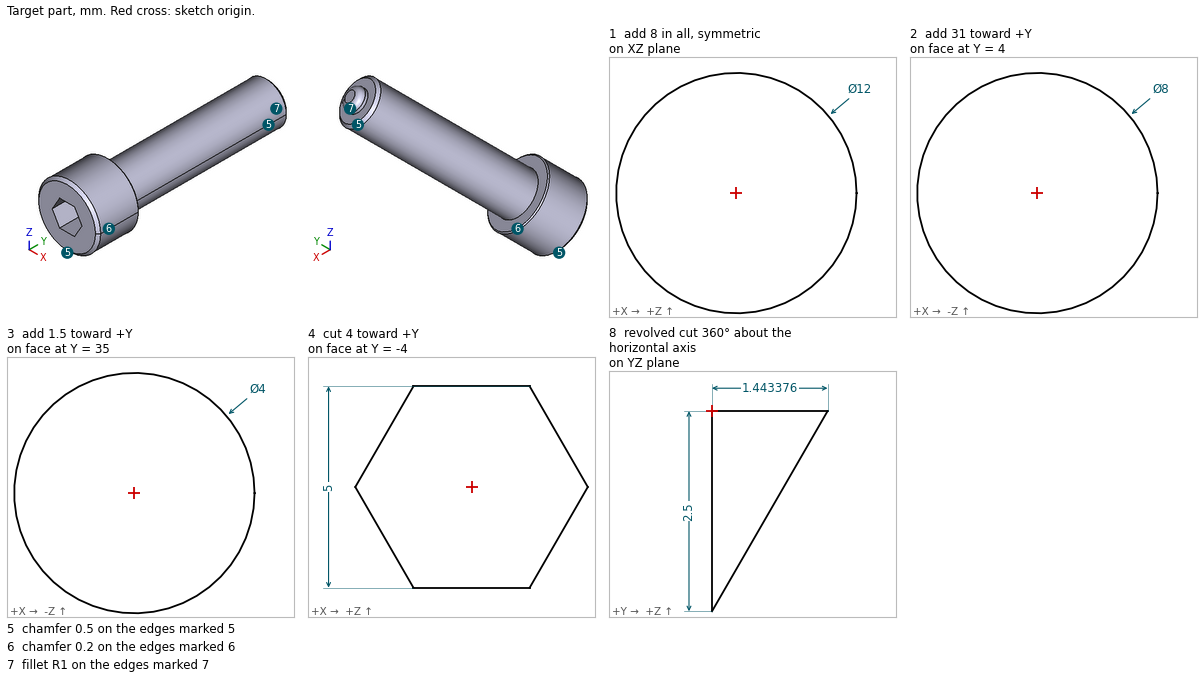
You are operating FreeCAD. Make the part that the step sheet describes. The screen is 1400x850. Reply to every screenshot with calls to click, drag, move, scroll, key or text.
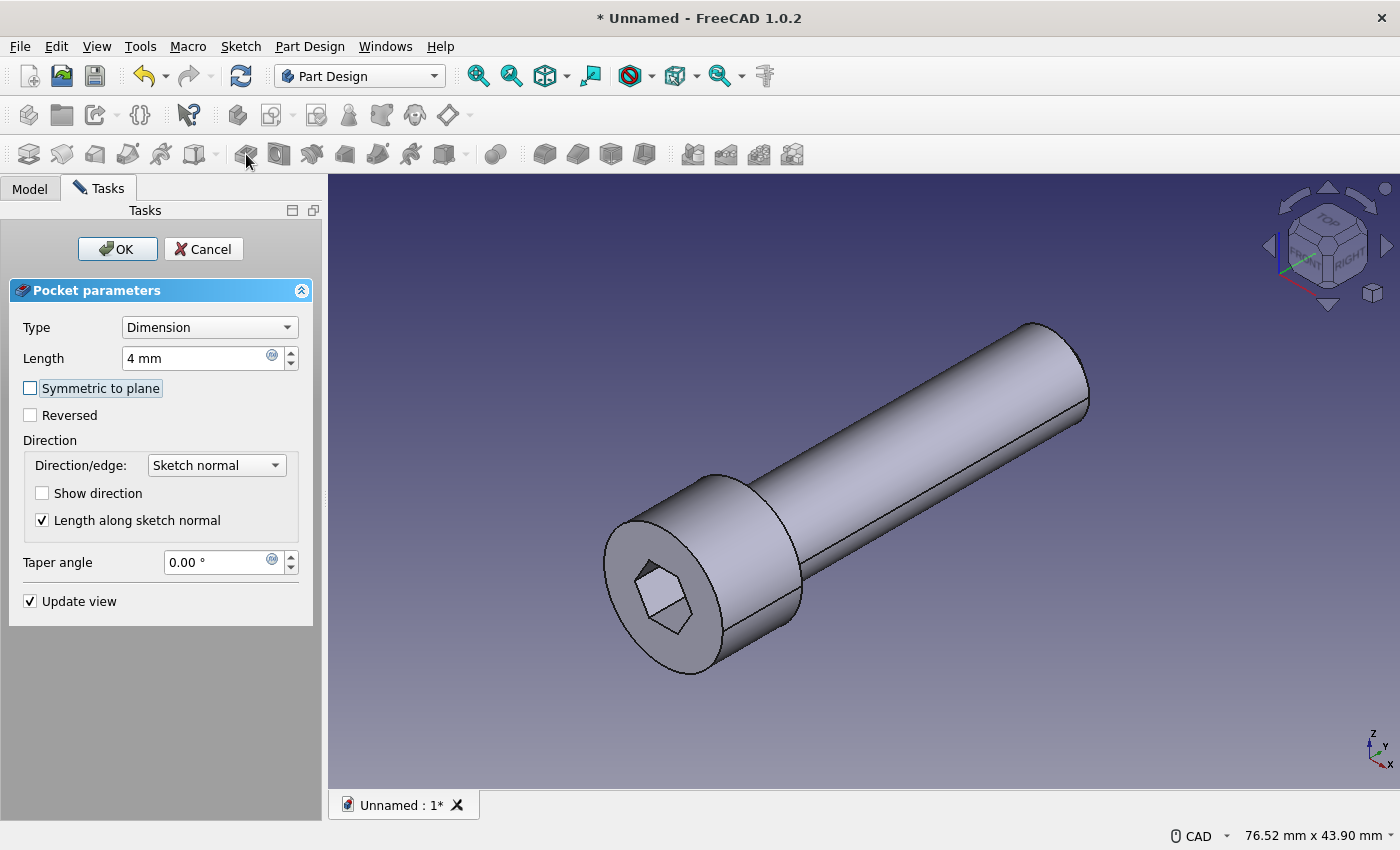
click(118, 249)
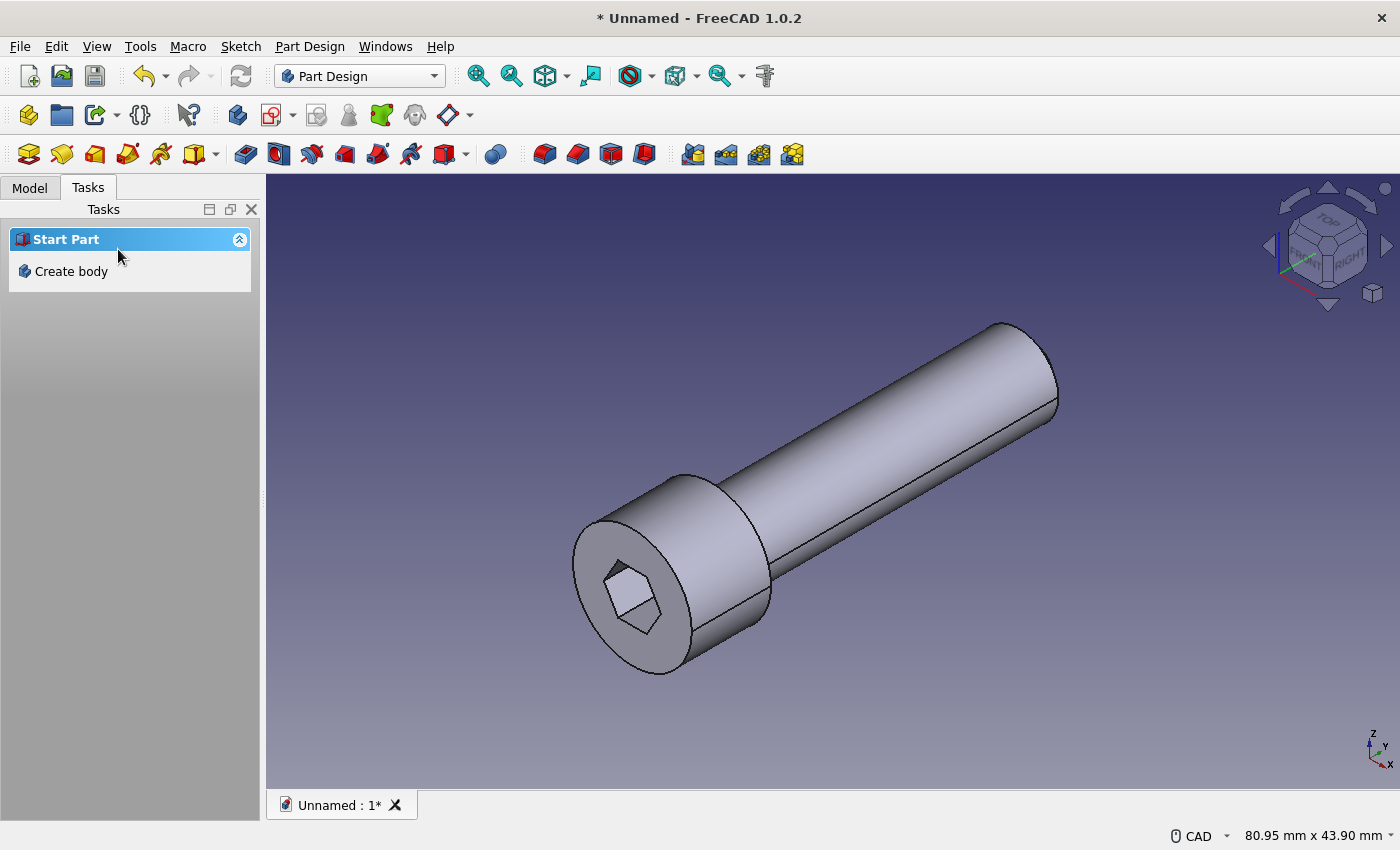
click(584, 528)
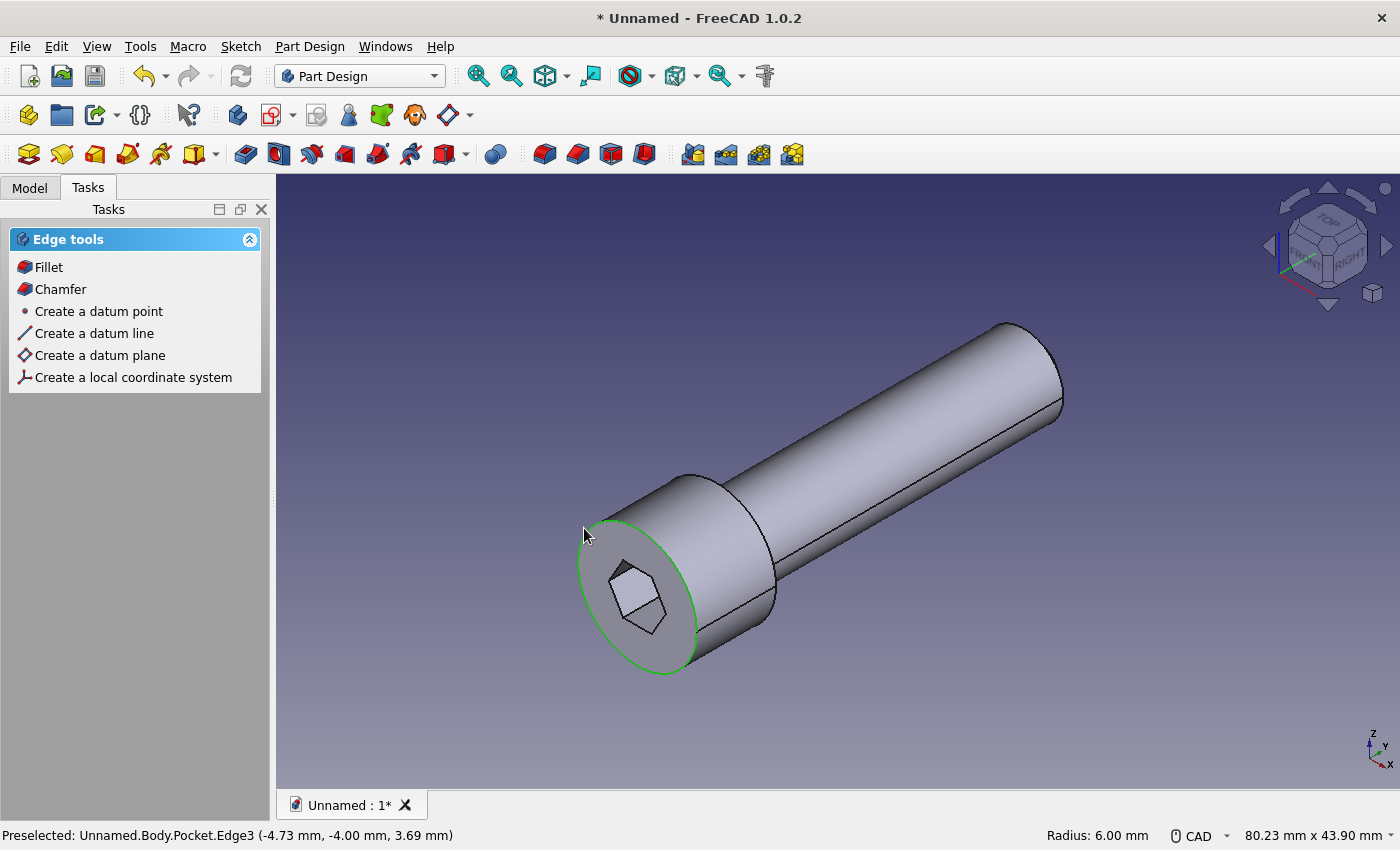
key(2)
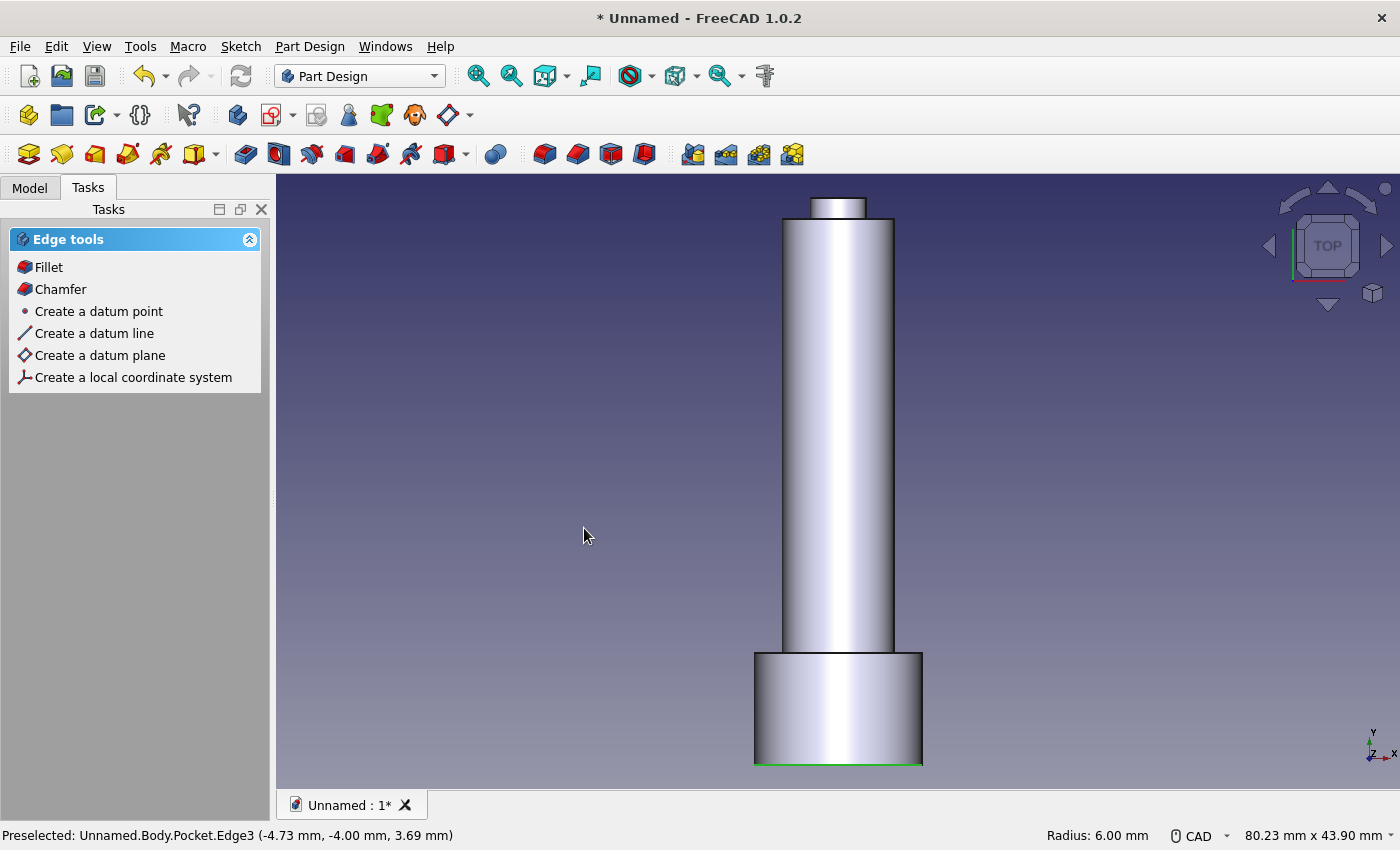
click(793, 218, ctrl)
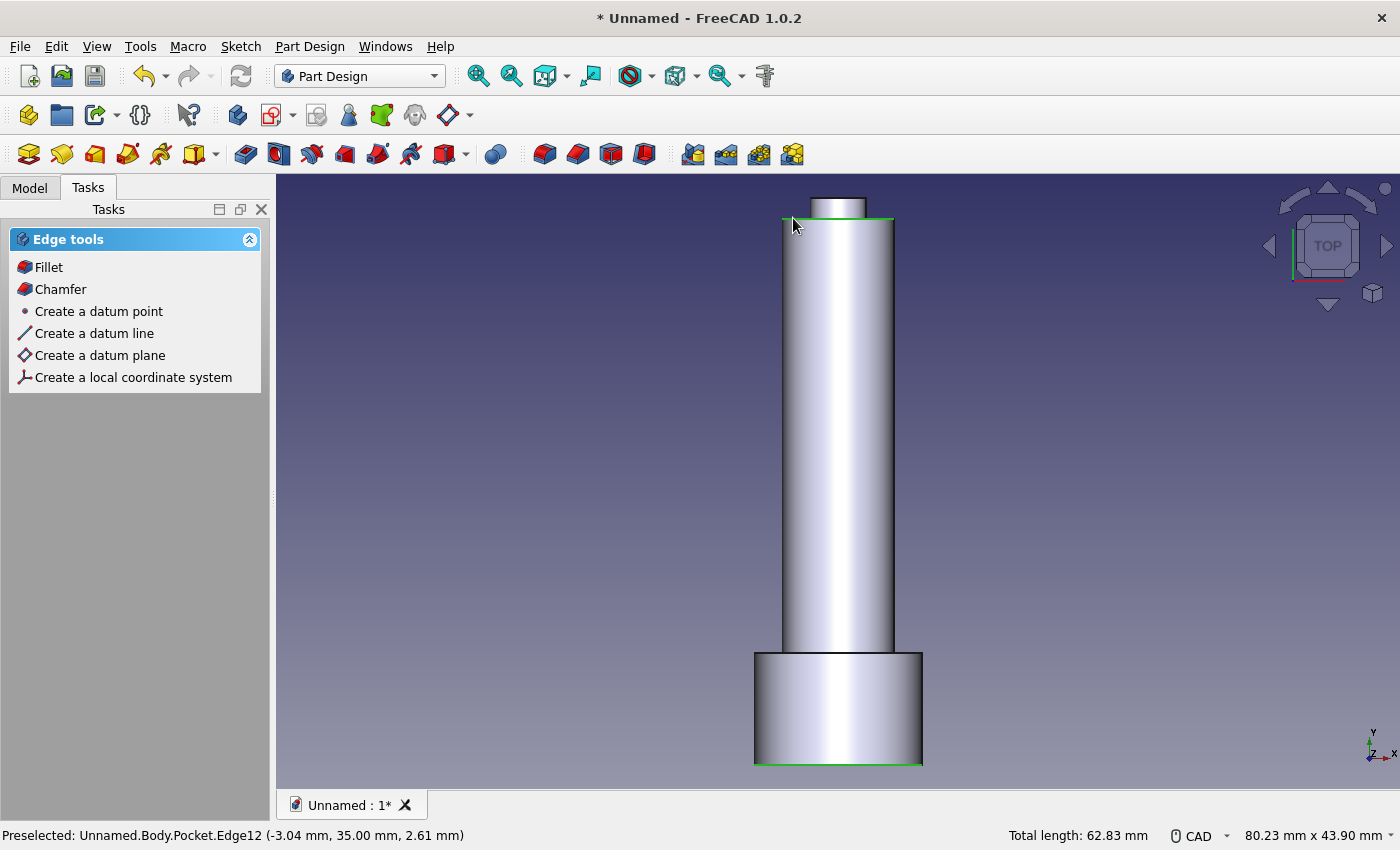
click(578, 154)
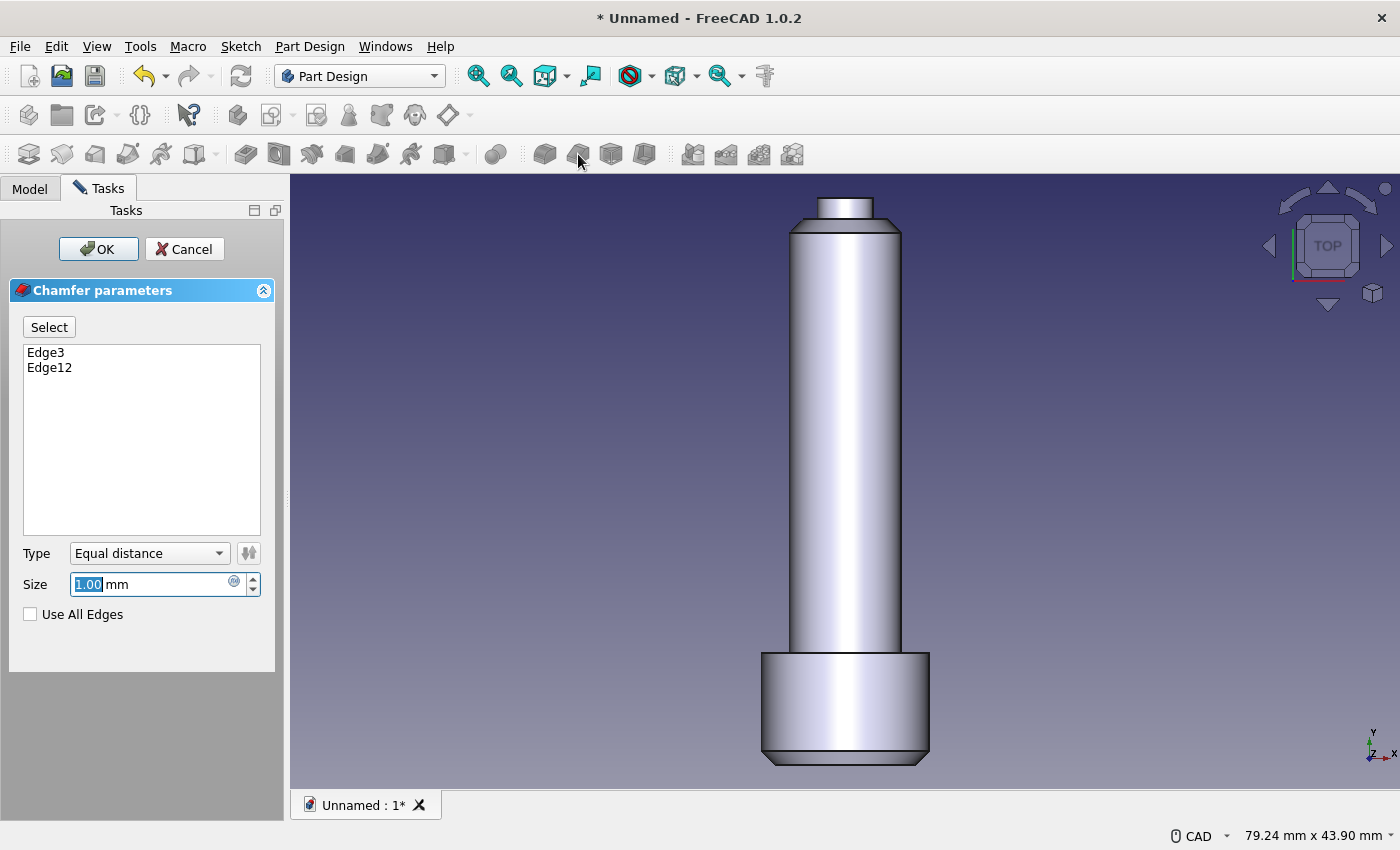
text(0.5)
key(Tab)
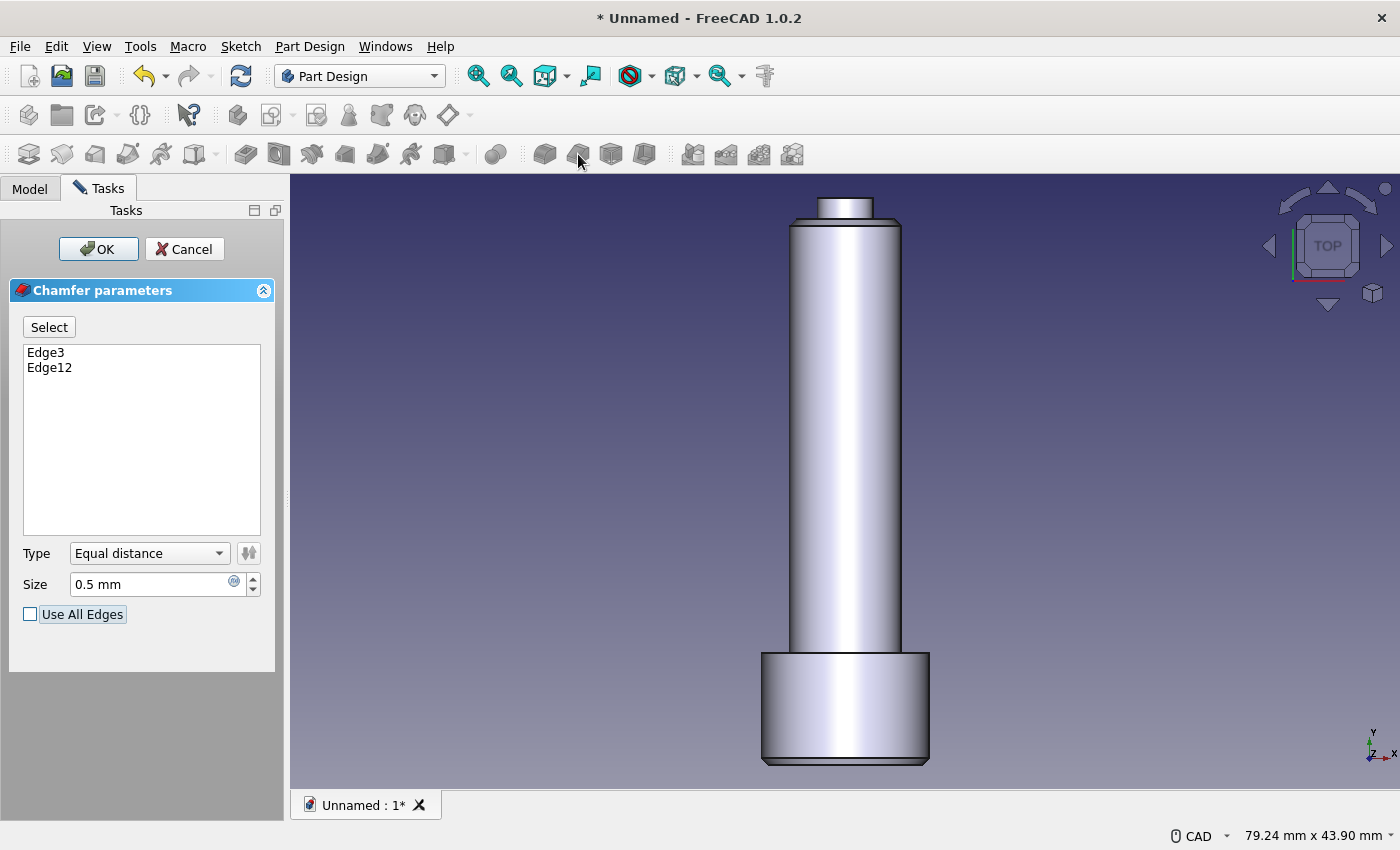
click(99, 249)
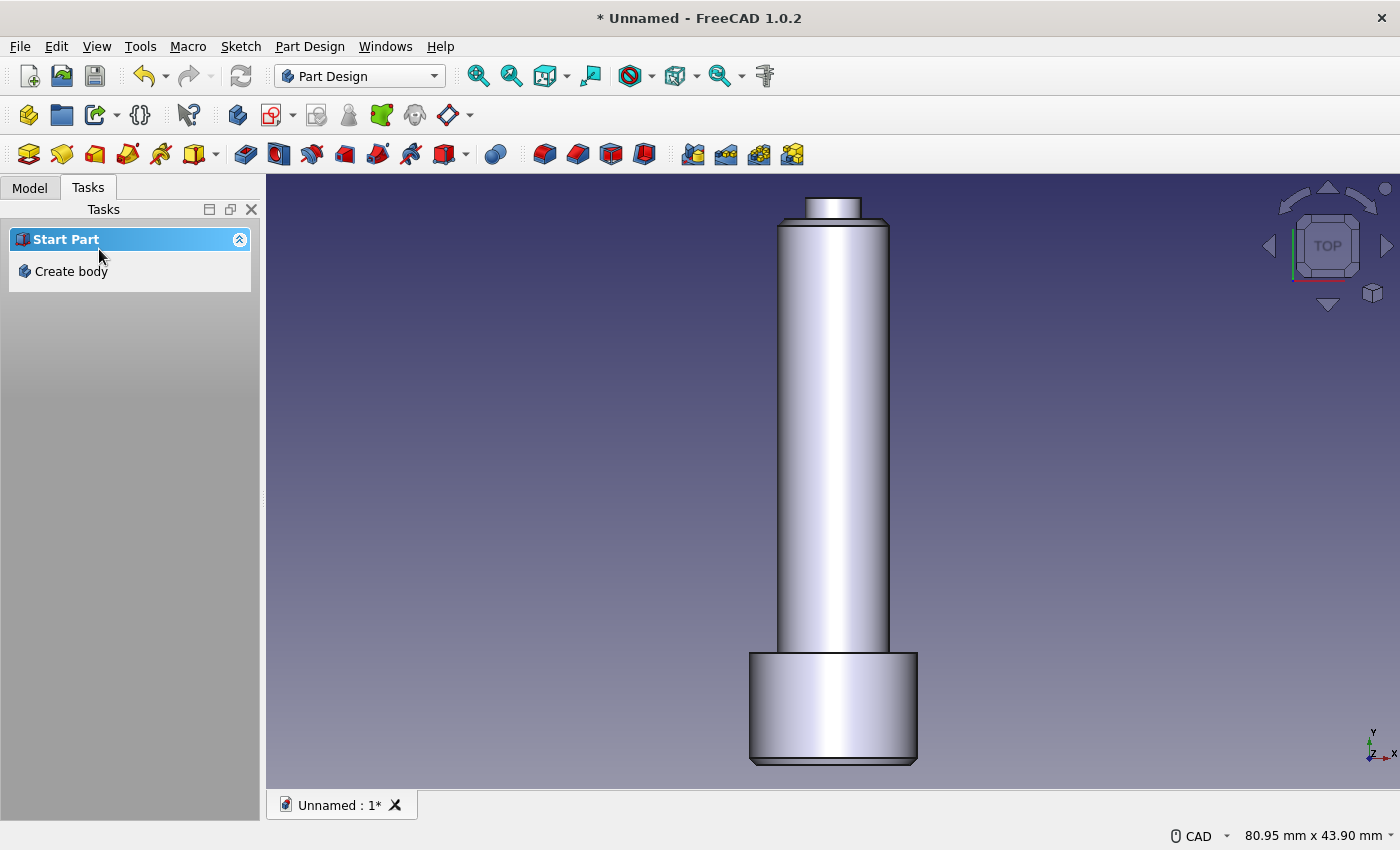
click(765, 652)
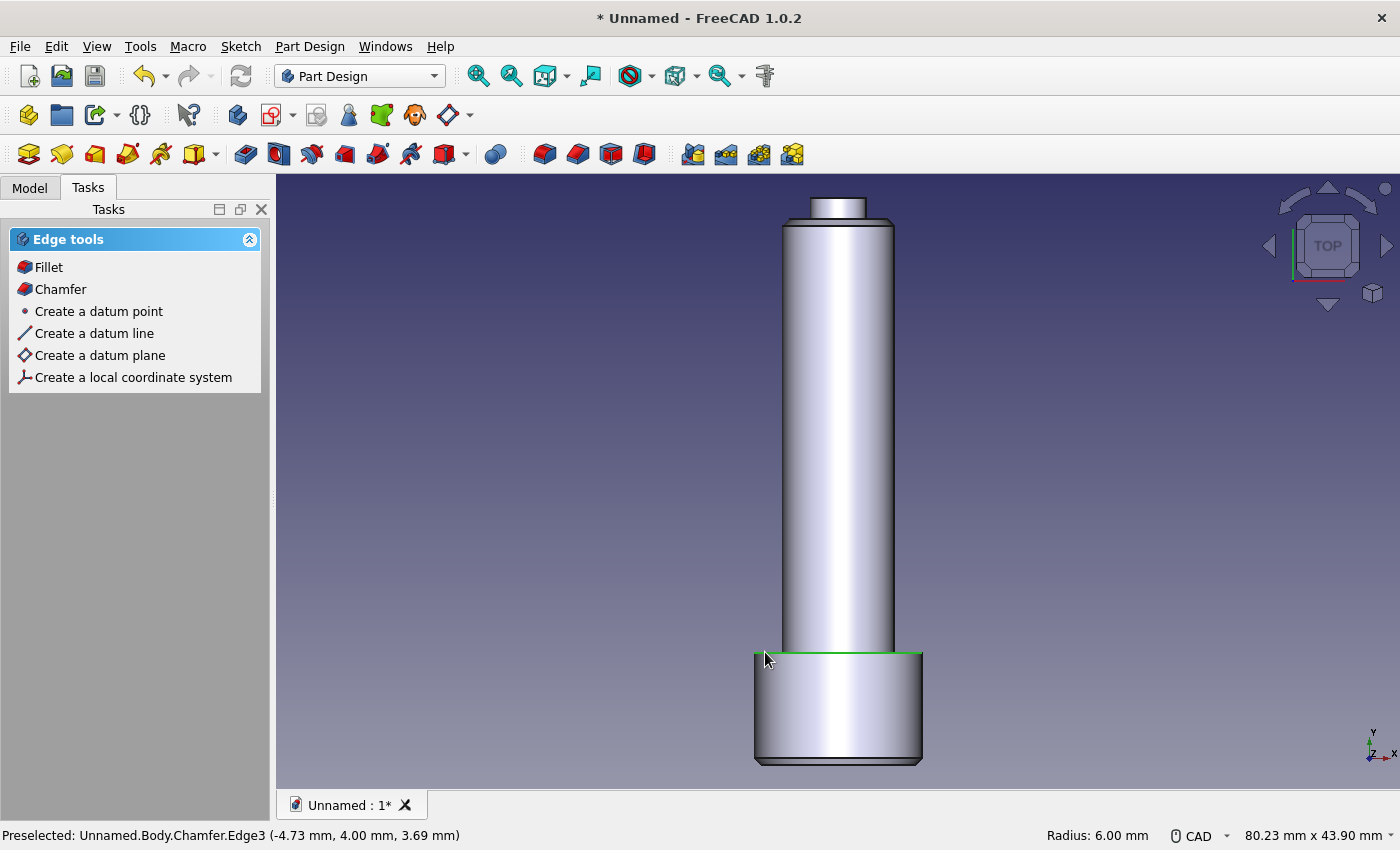
click(578, 154)